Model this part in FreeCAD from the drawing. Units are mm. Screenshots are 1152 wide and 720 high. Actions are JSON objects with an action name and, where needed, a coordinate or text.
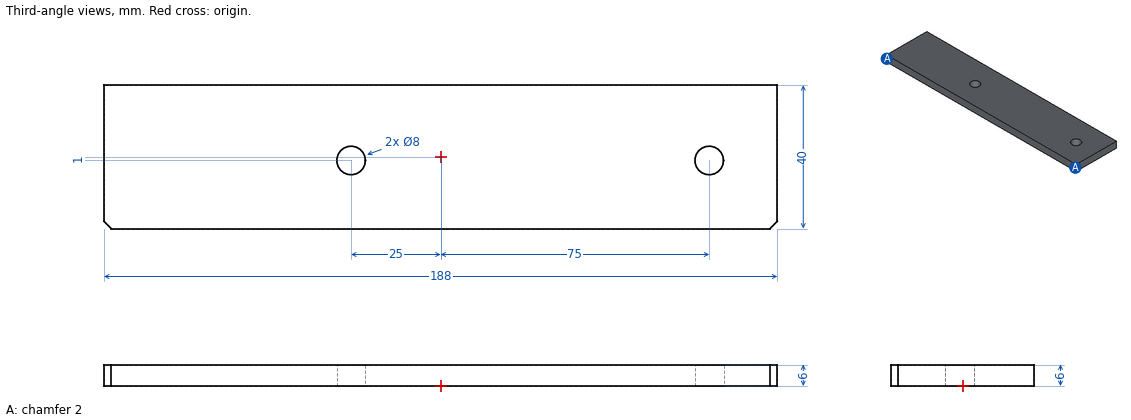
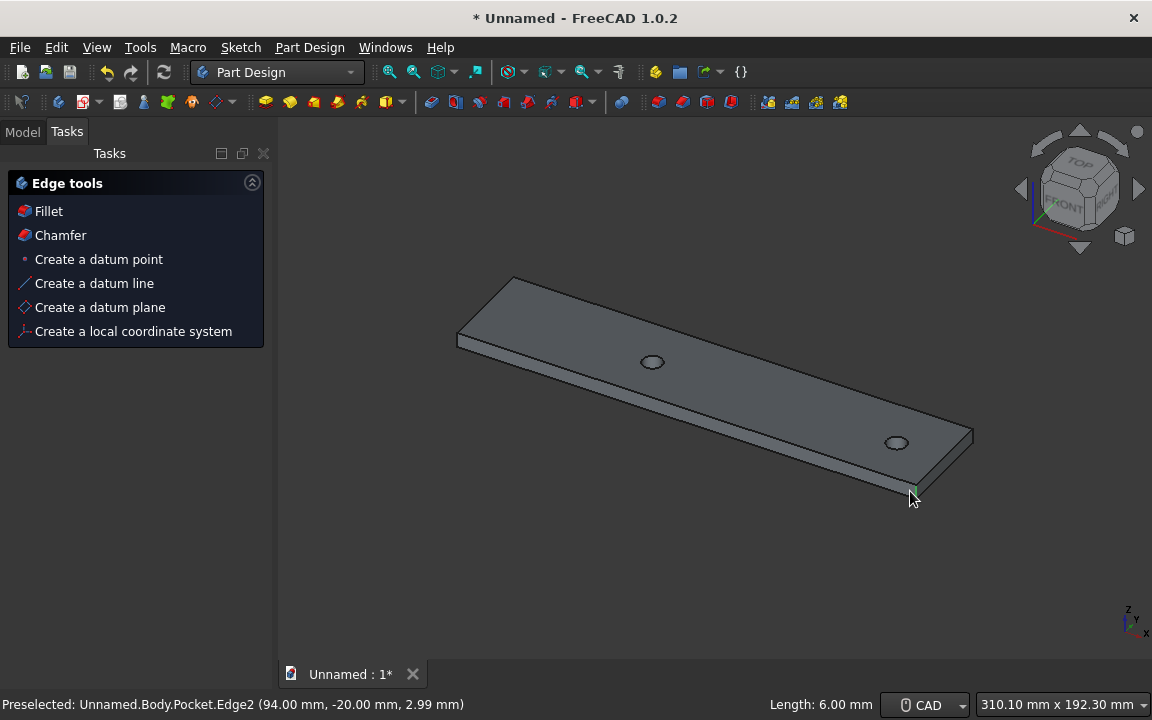
{"action": "scroll", "coordinate": [457, 339], "scroll_direction": "up", "scroll_amount": 5}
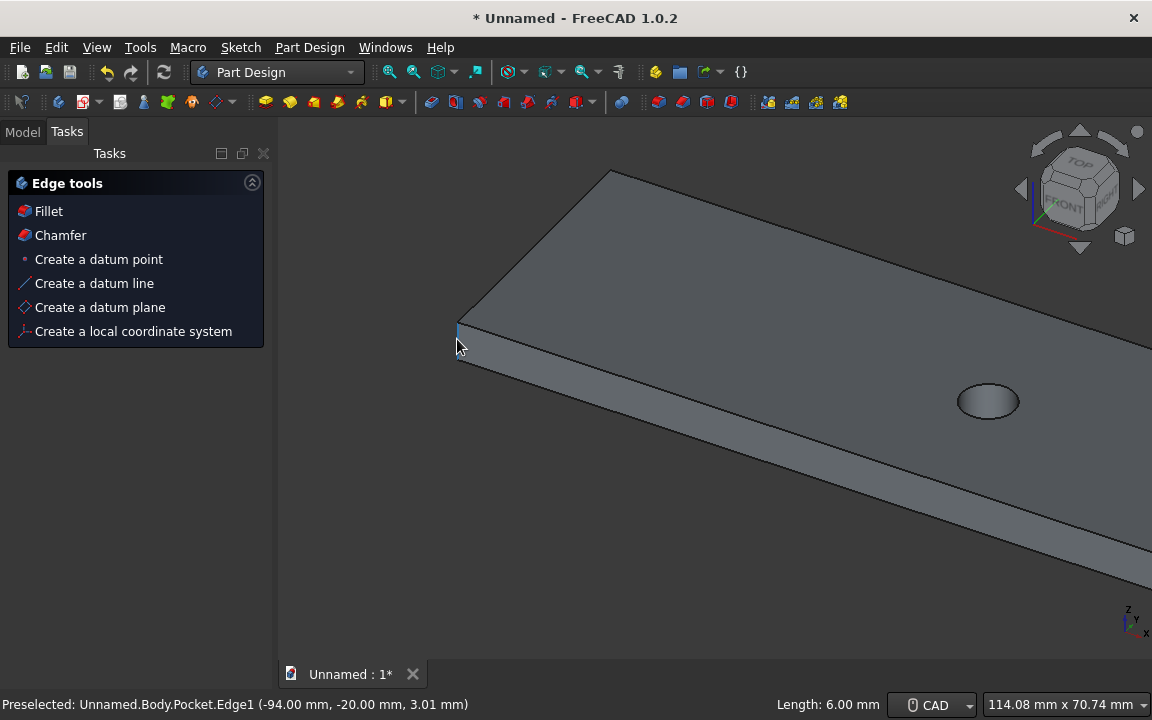
{"action": "key", "text": "v f"}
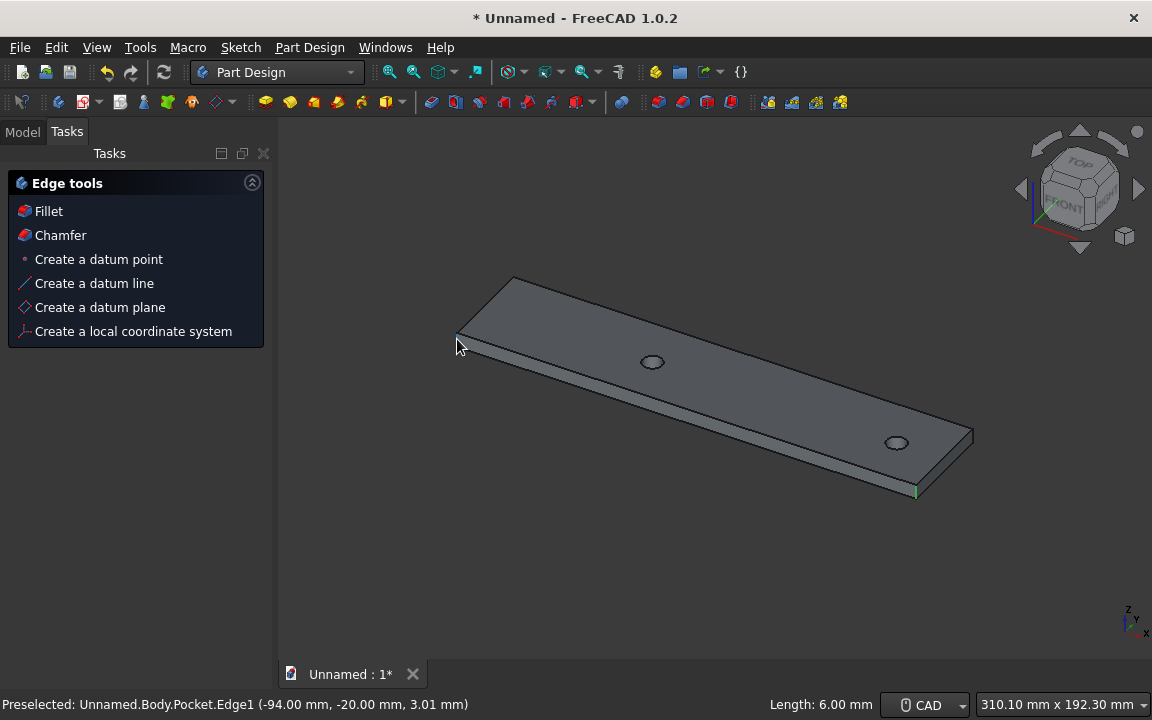
{"action": "key", "text": "0"}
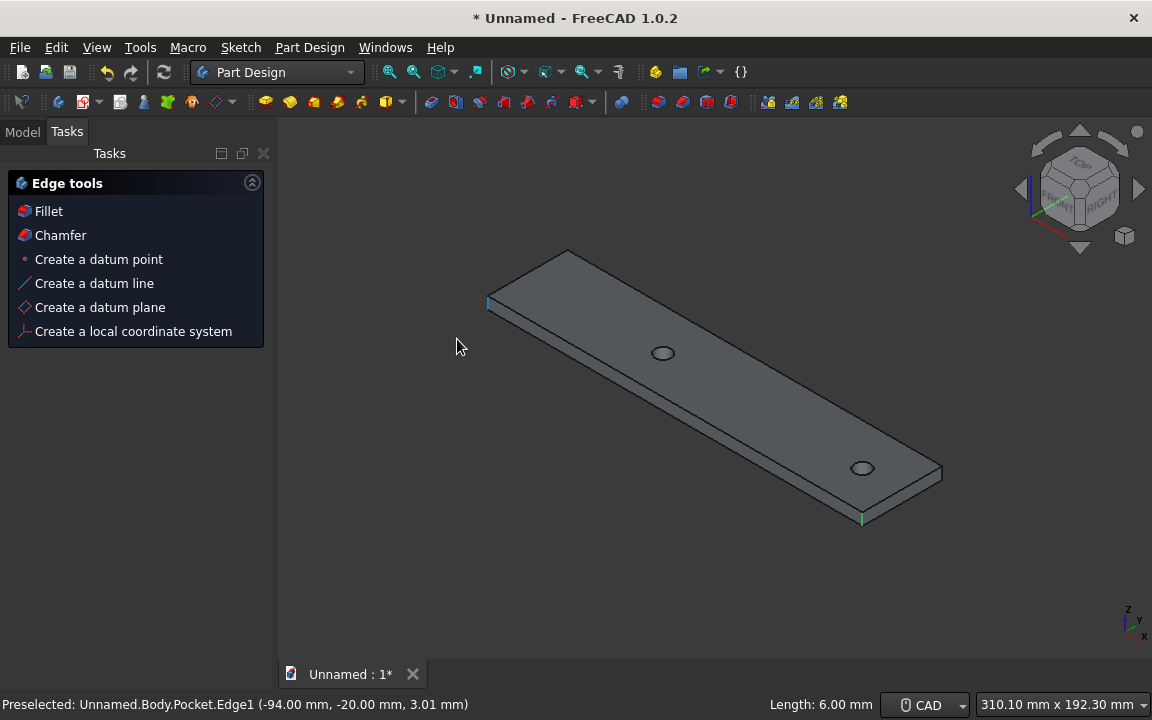
{"action": "scroll", "coordinate": [488, 302], "scroll_direction": "up", "scroll_amount": 5}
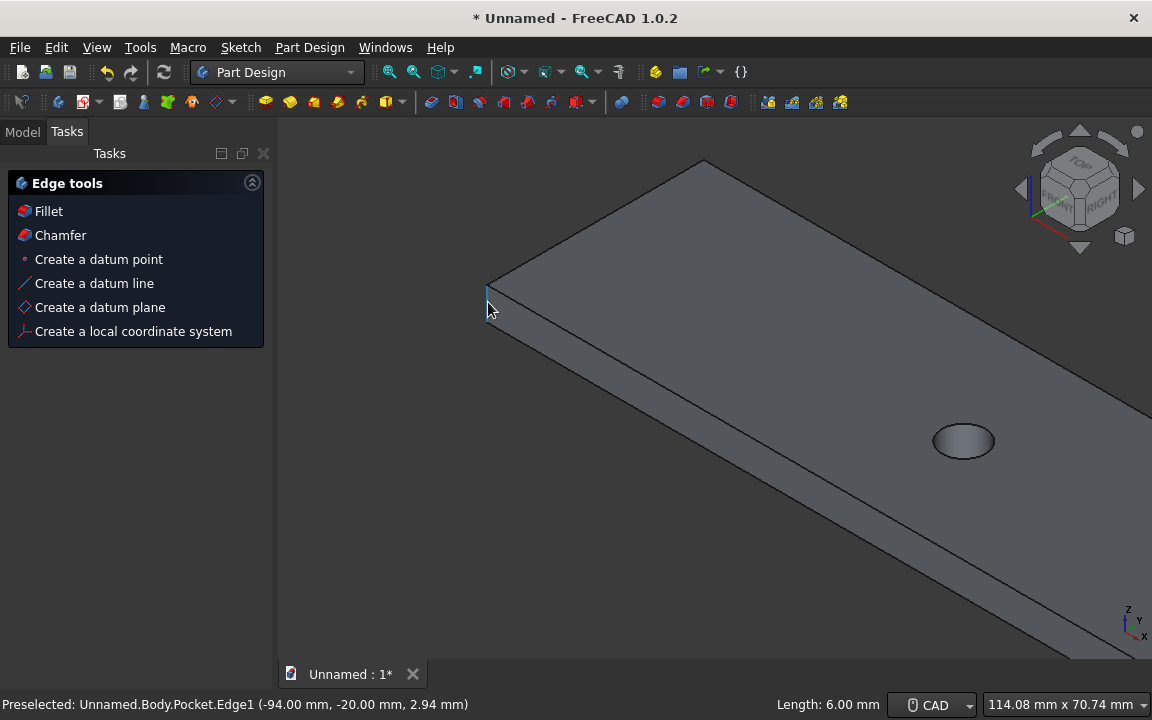
{"action": "left_click", "coordinate": [390, 72]}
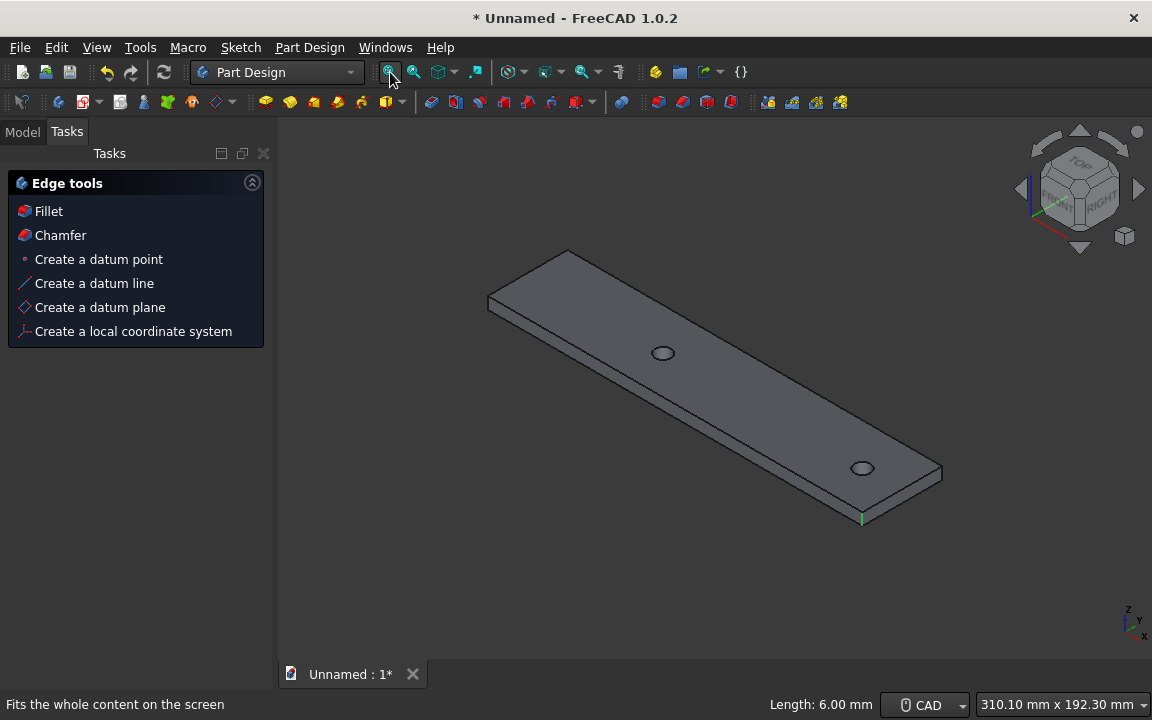
{"action": "key", "text": "2"}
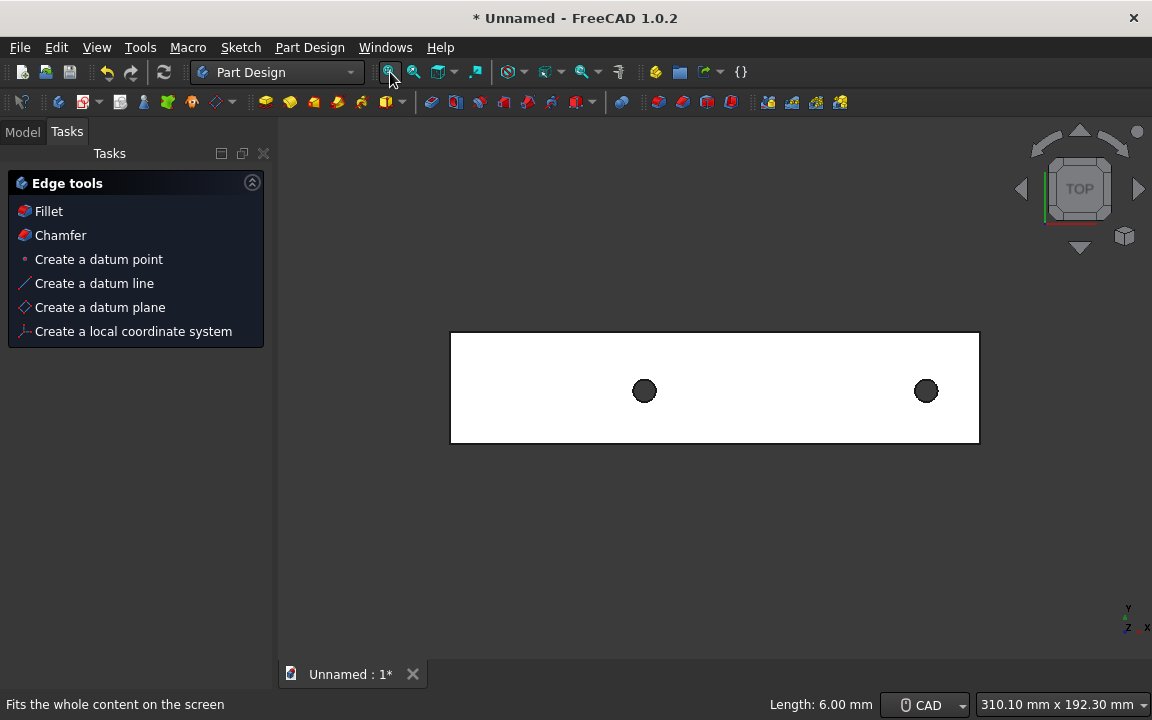
{"action": "scroll", "coordinate": [450, 443], "scroll_direction": "up", "scroll_amount": 5}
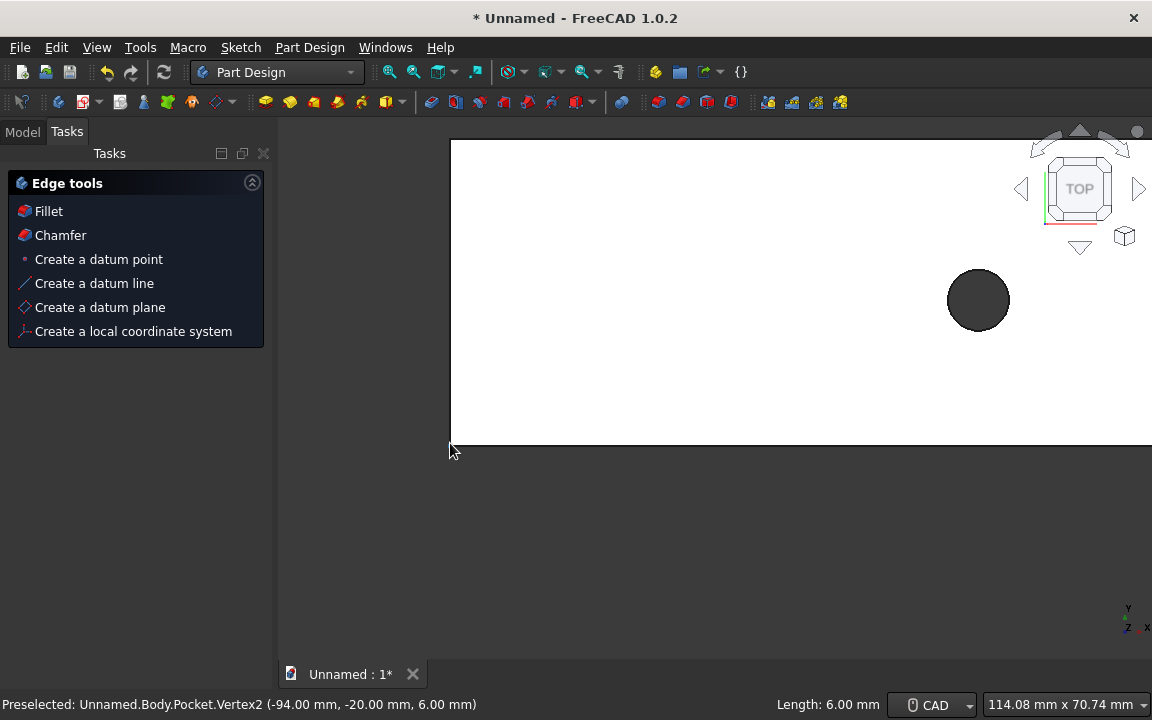
{"action": "left_click", "coordinate": [390, 72]}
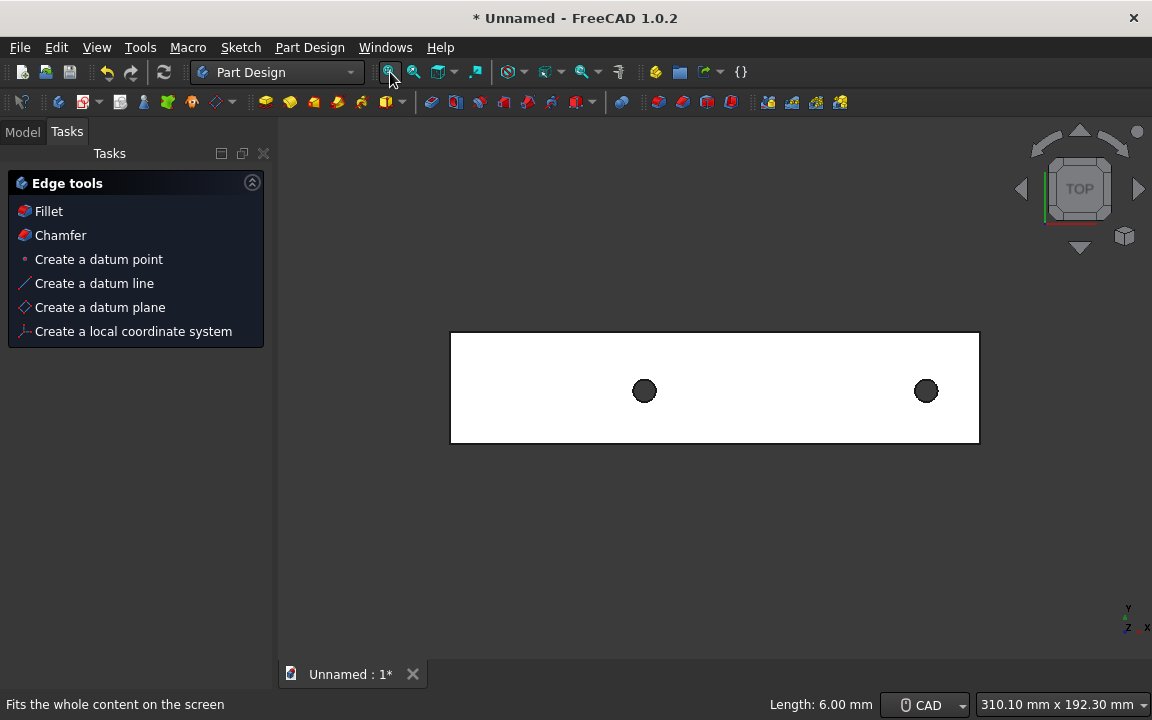
{"action": "key", "text": "1"}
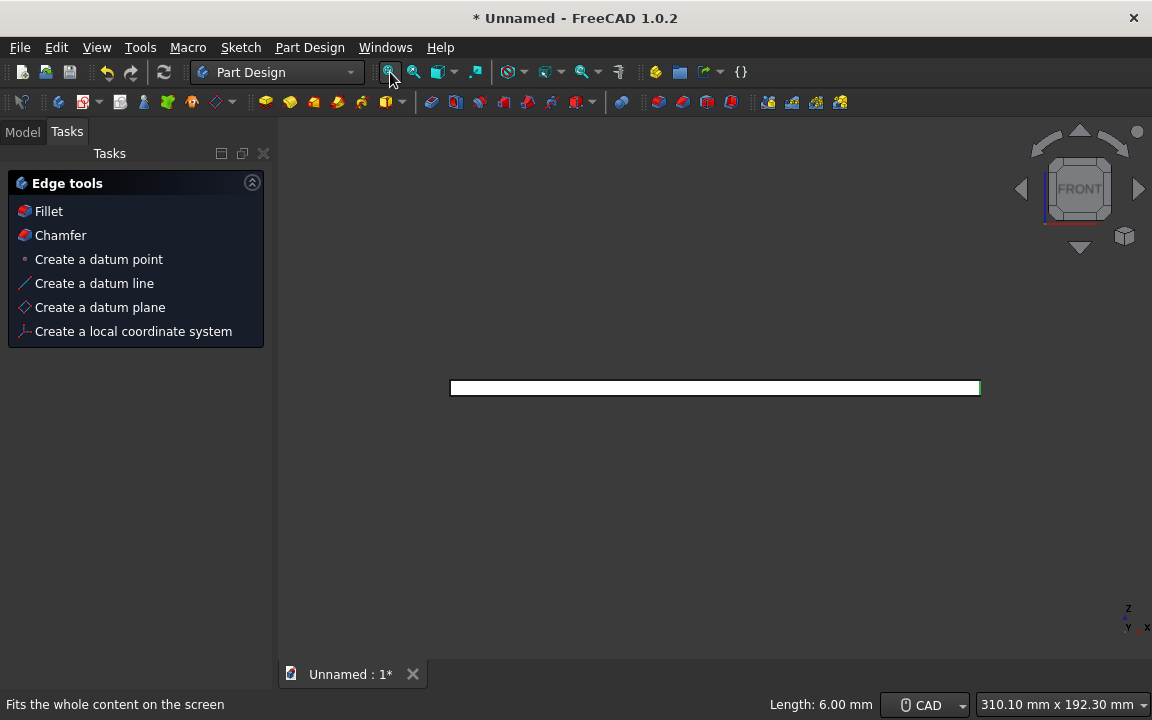
{"action": "left_click", "coordinate": [450, 387], "text": "ctrl"}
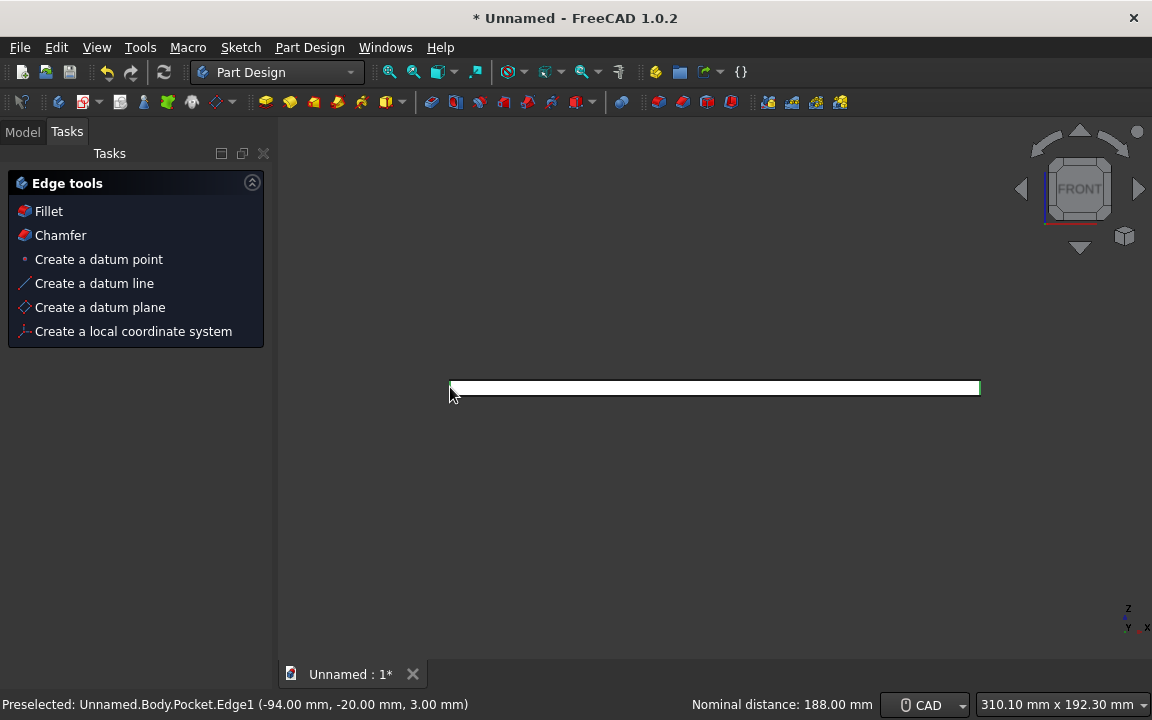
{"action": "left_click", "coordinate": [684, 102]}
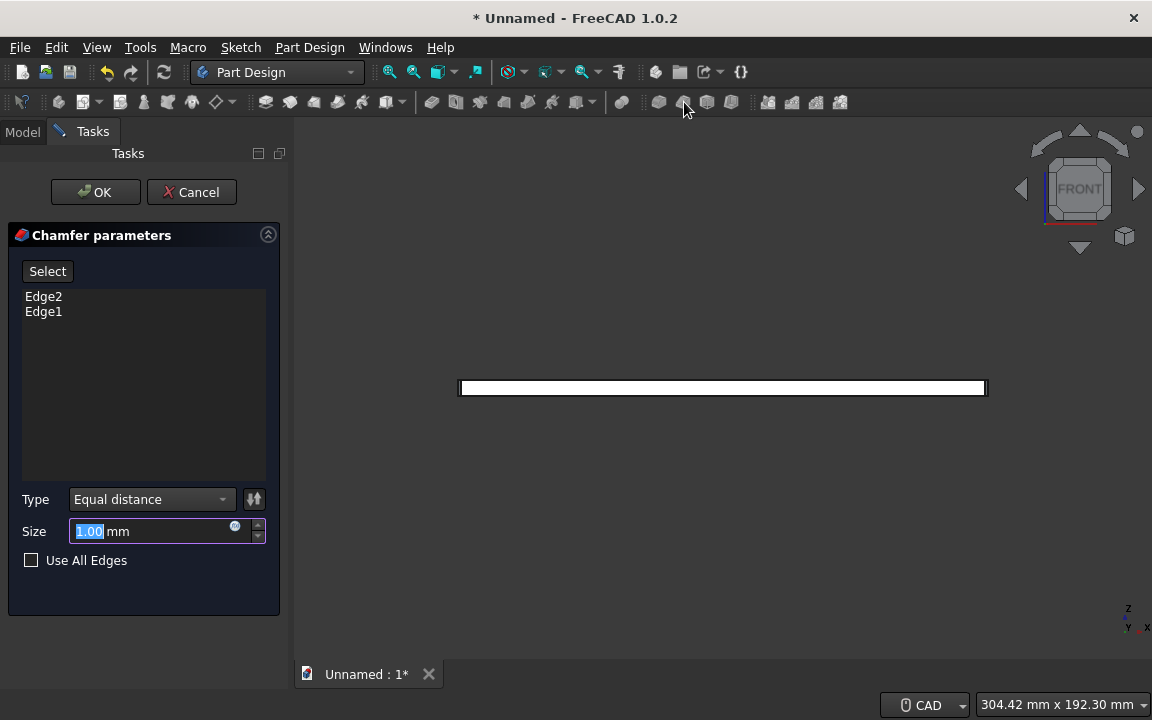
{"action": "type", "text": "2"}
{"action": "key", "text": "Tab"}